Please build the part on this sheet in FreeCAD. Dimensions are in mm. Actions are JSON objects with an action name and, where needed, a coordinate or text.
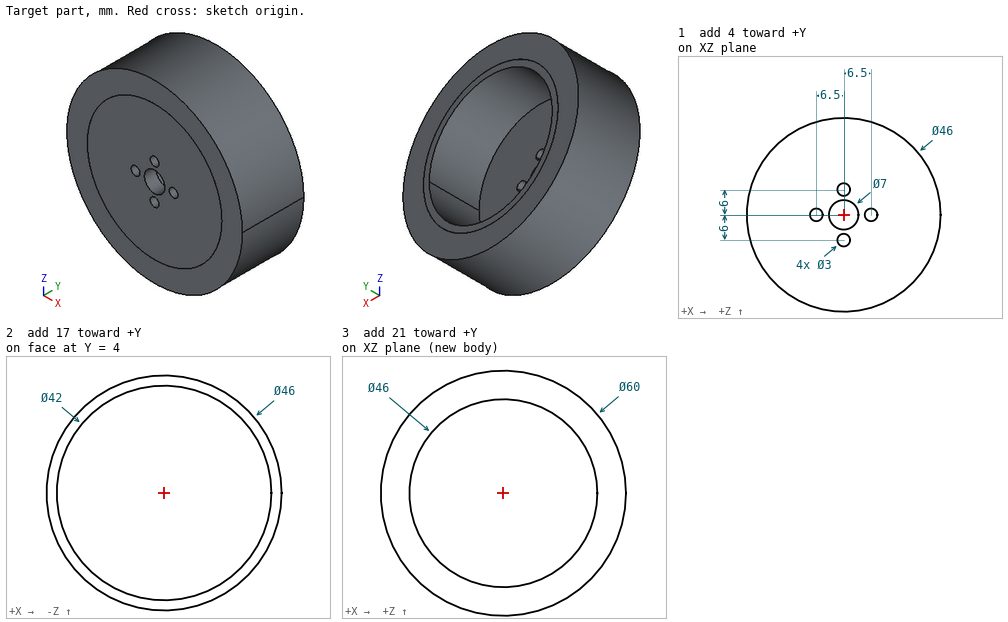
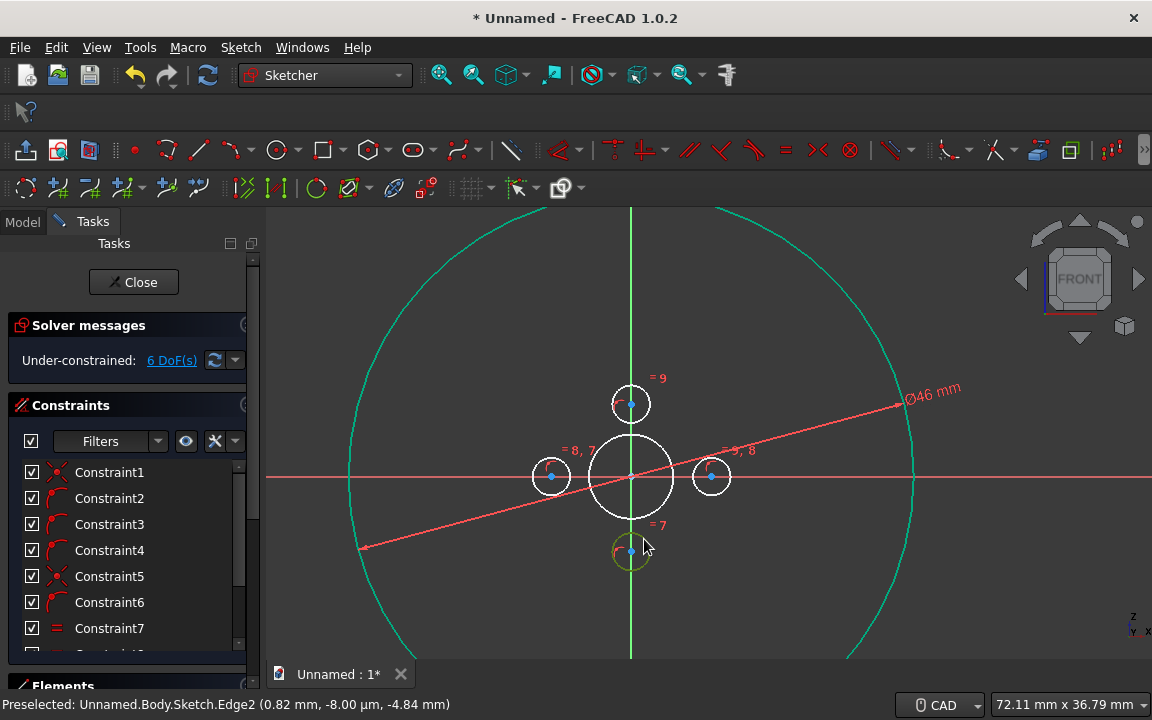
{"action": "left_click", "coordinate": [582, 150]}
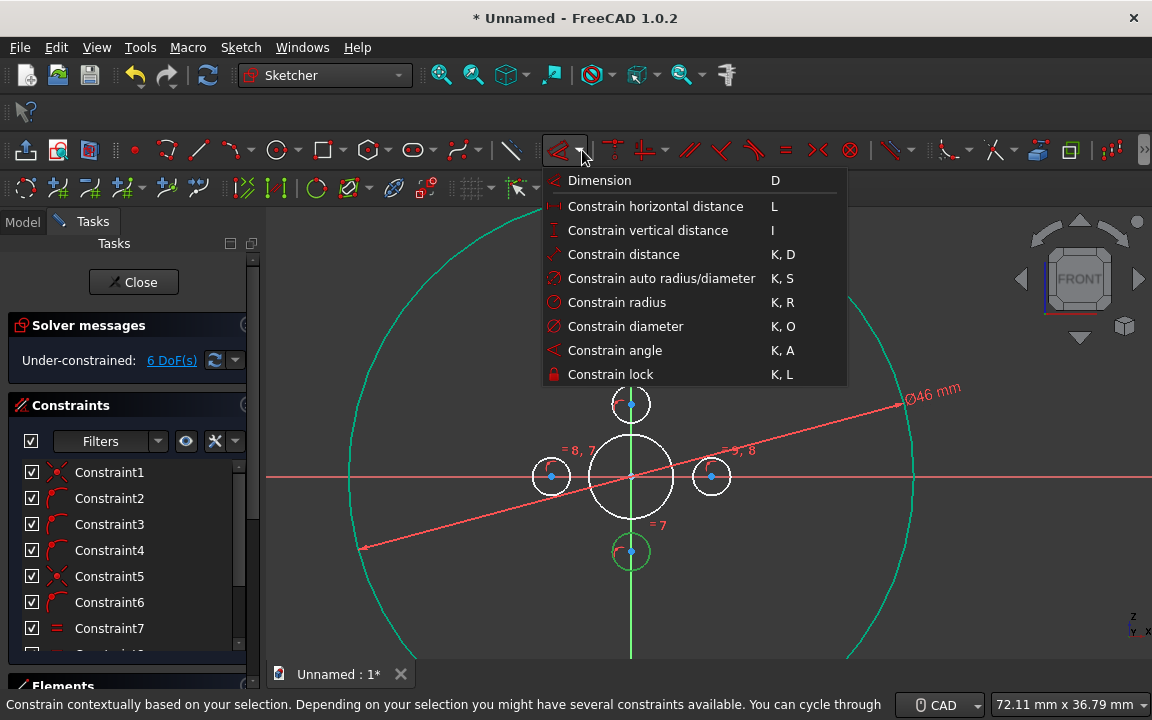
{"action": "left_click", "coordinate": [695, 326]}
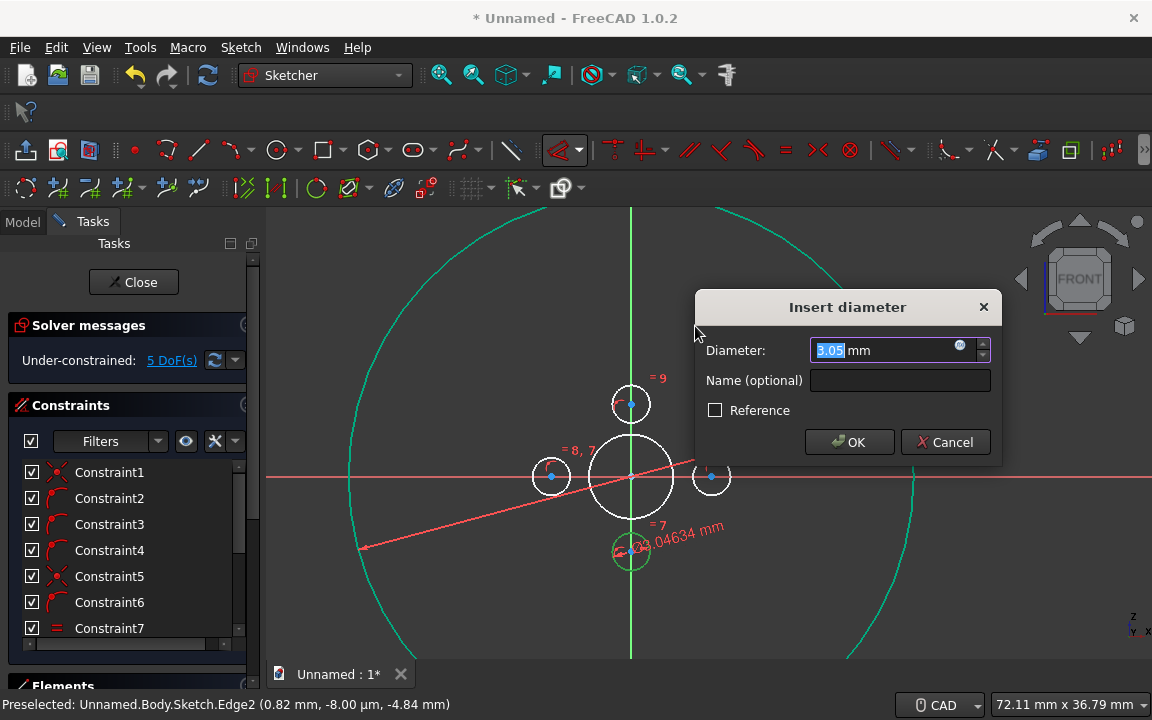
{"action": "type", "text": "3"}
{"action": "key", "text": "Return"}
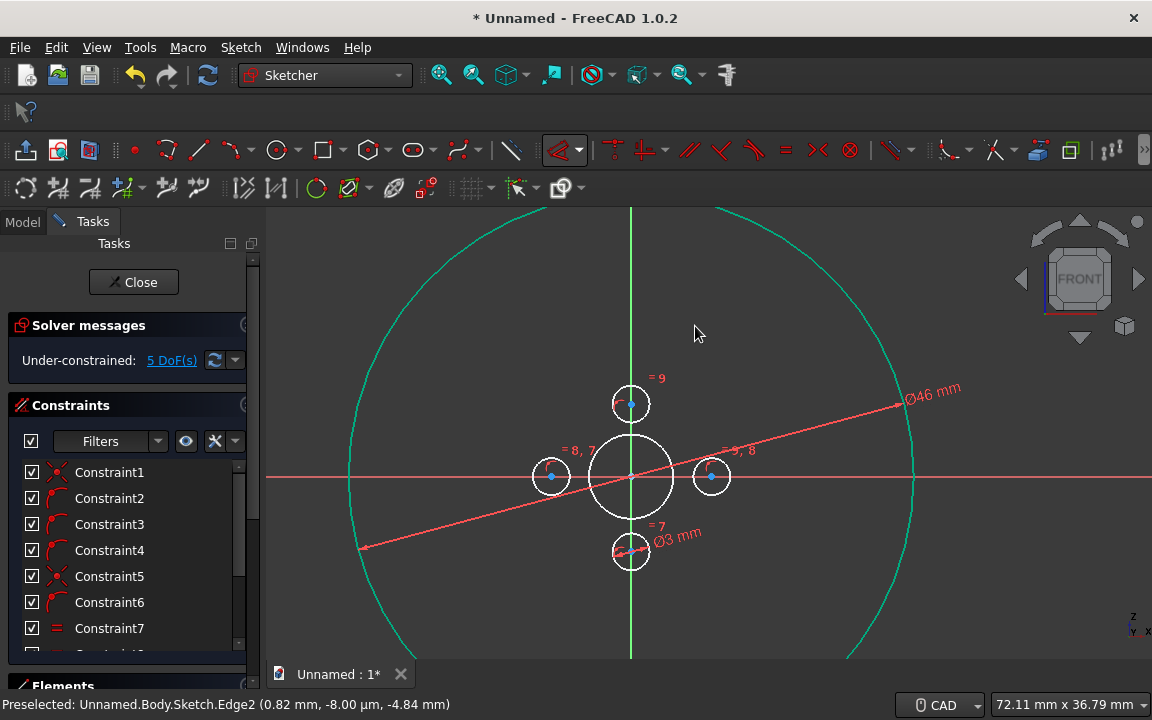
{"action": "left_click", "coordinate": [661, 447]}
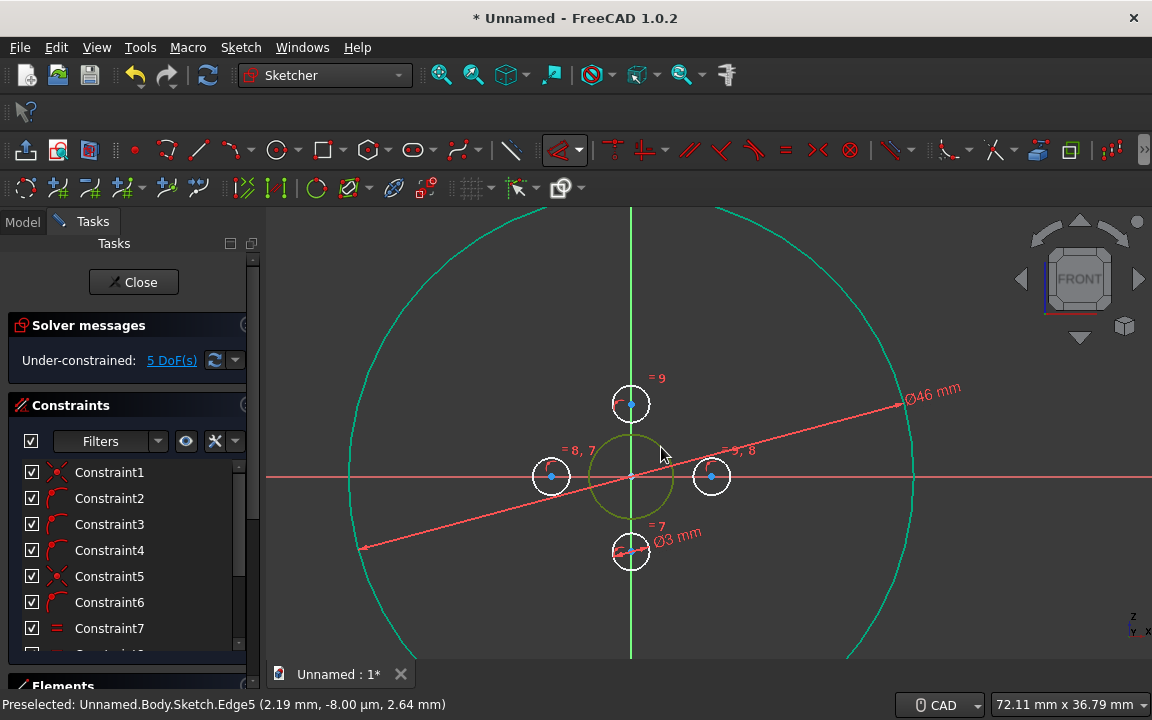
{"action": "key", "text": "k o"}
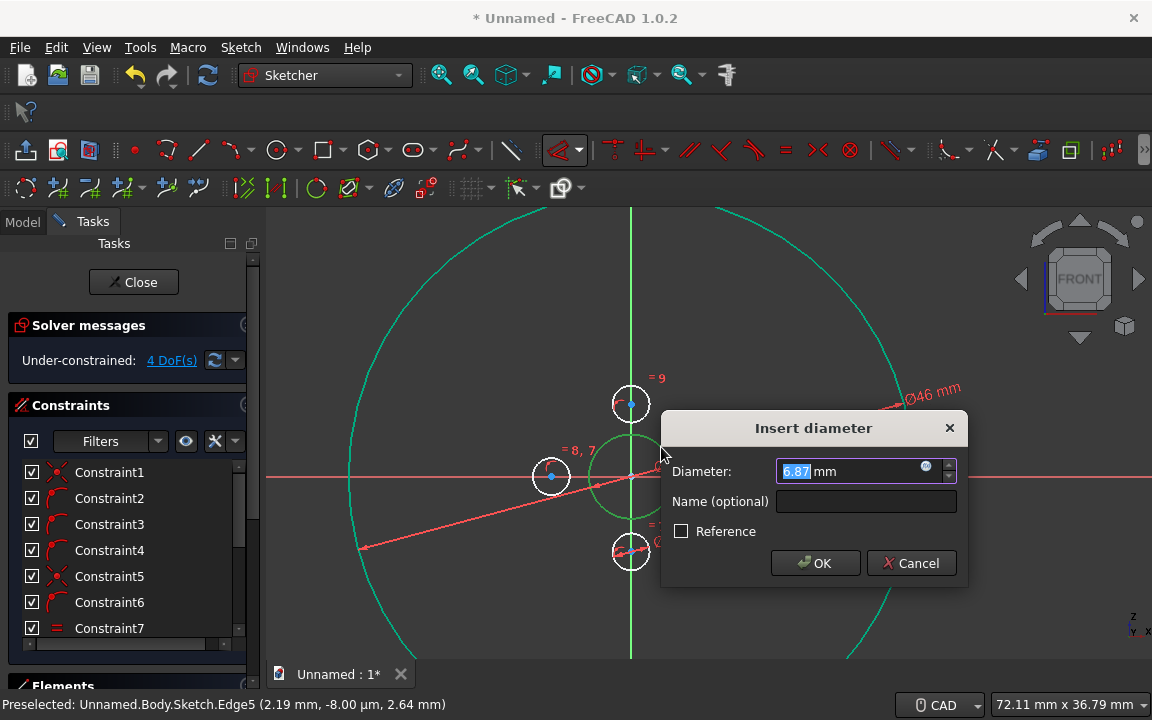
{"action": "type", "text": "7"}
{"action": "key", "text": "Return"}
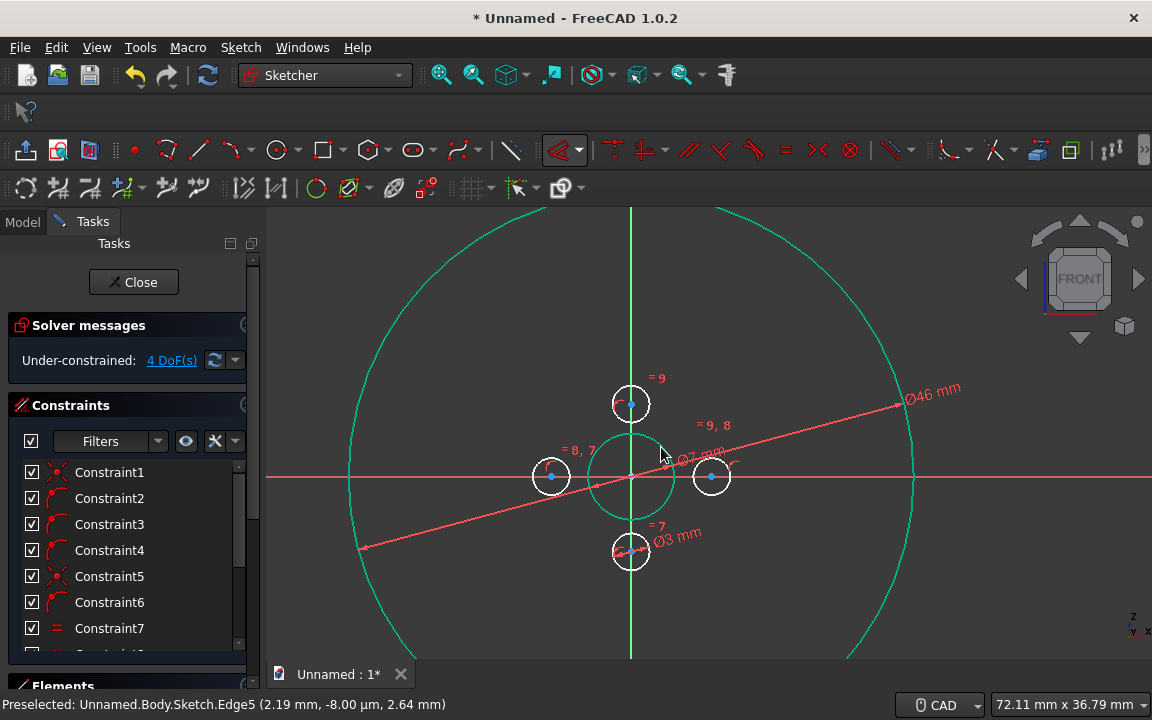
{"action": "left_click", "coordinate": [631, 552]}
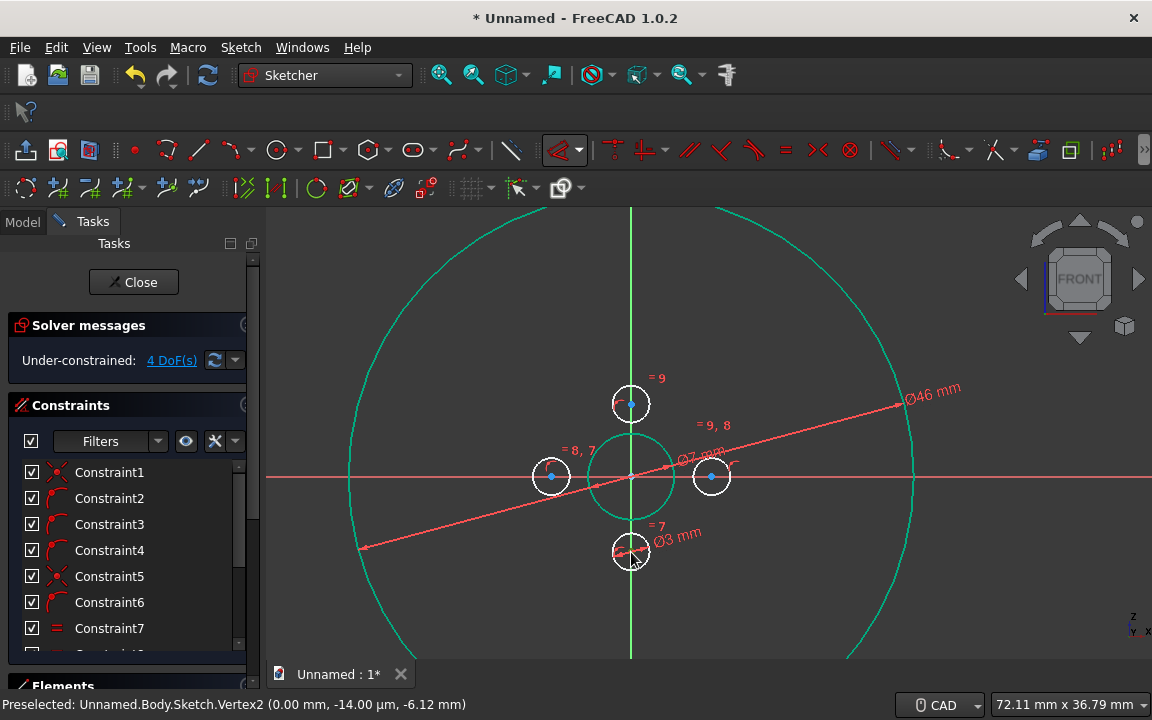
{"action": "key", "text": "i"}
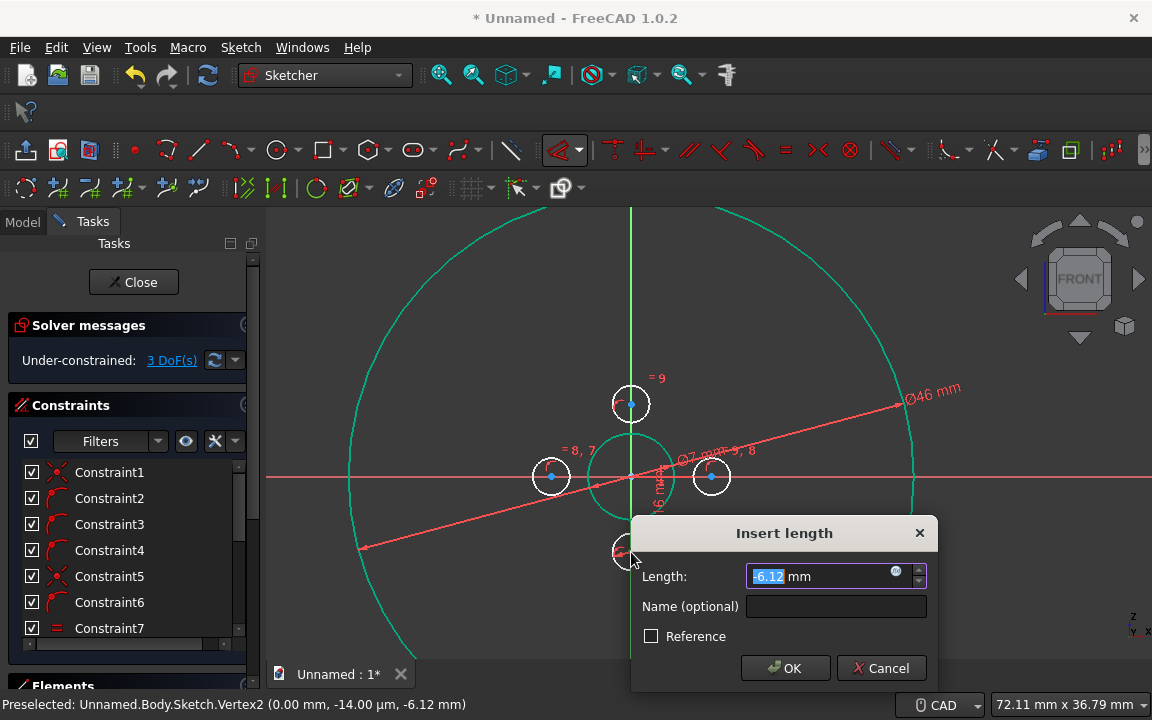
{"action": "type", "text": "-6"}
{"action": "key", "text": "Return"}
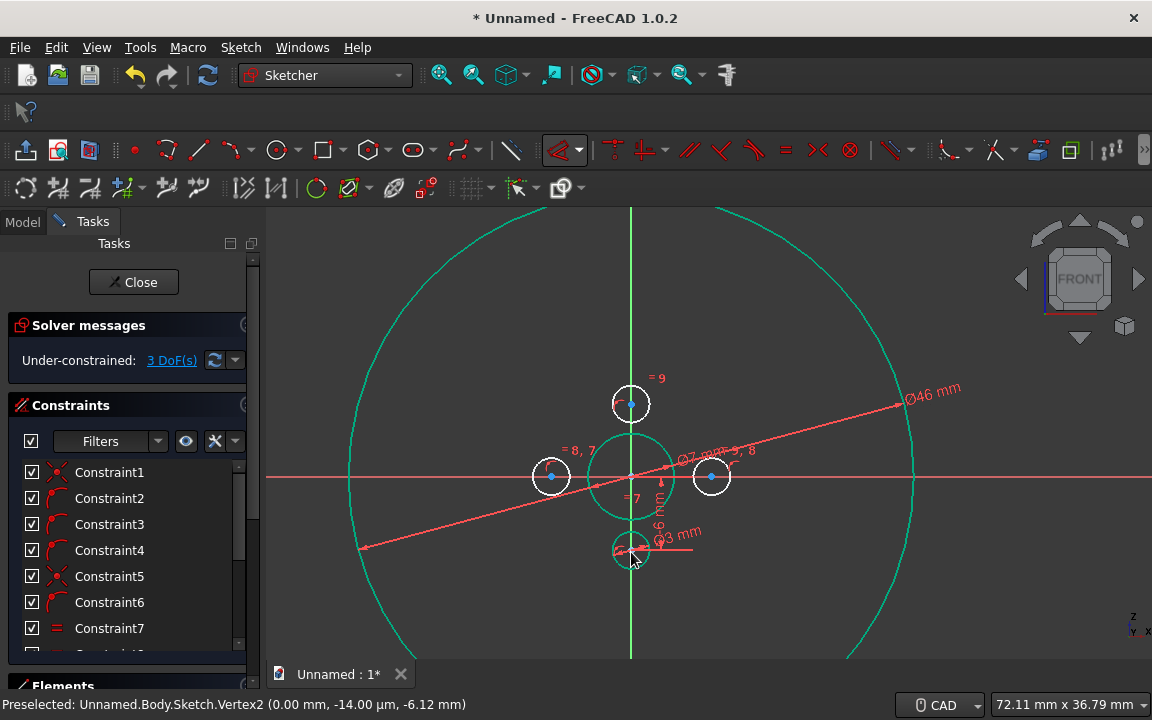
{"action": "left_click", "coordinate": [631, 404]}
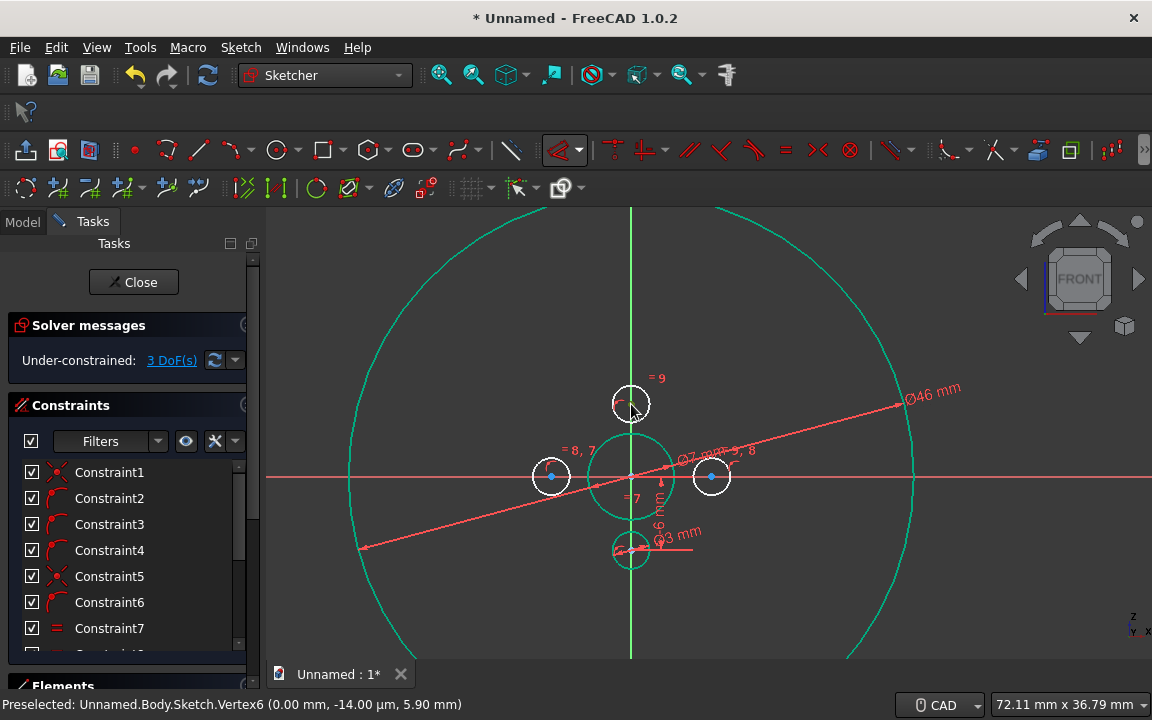
{"action": "left_click", "coordinate": [582, 150]}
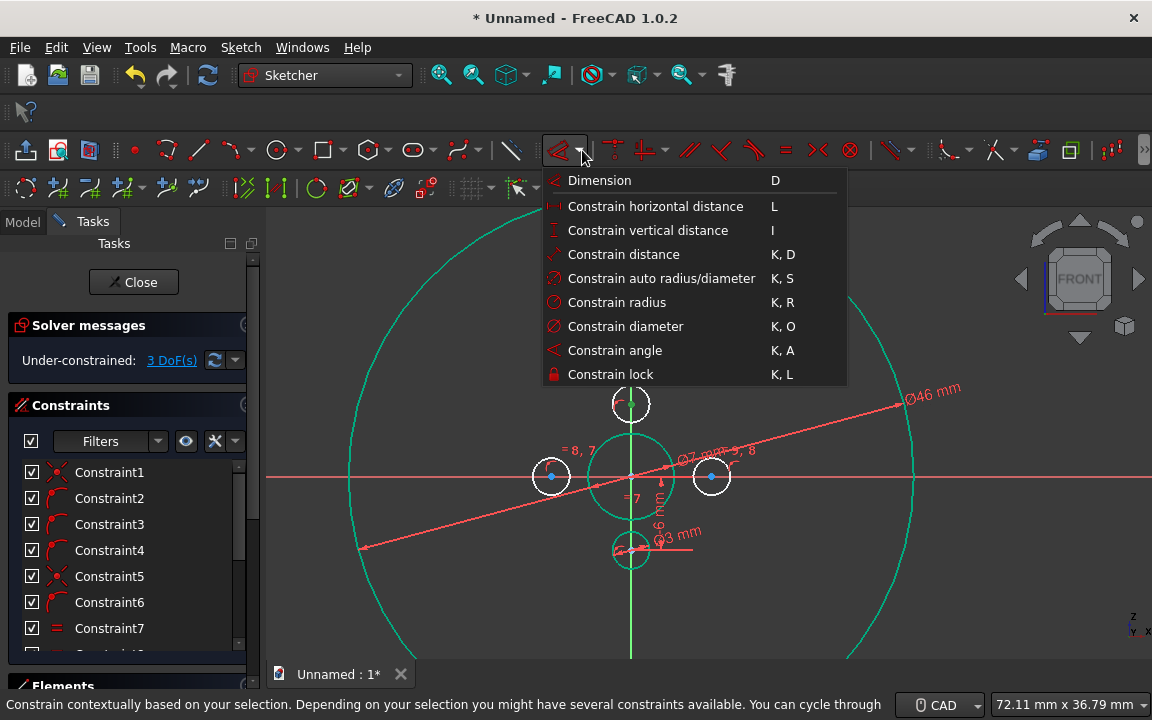
{"action": "left_click", "coordinate": [695, 230]}